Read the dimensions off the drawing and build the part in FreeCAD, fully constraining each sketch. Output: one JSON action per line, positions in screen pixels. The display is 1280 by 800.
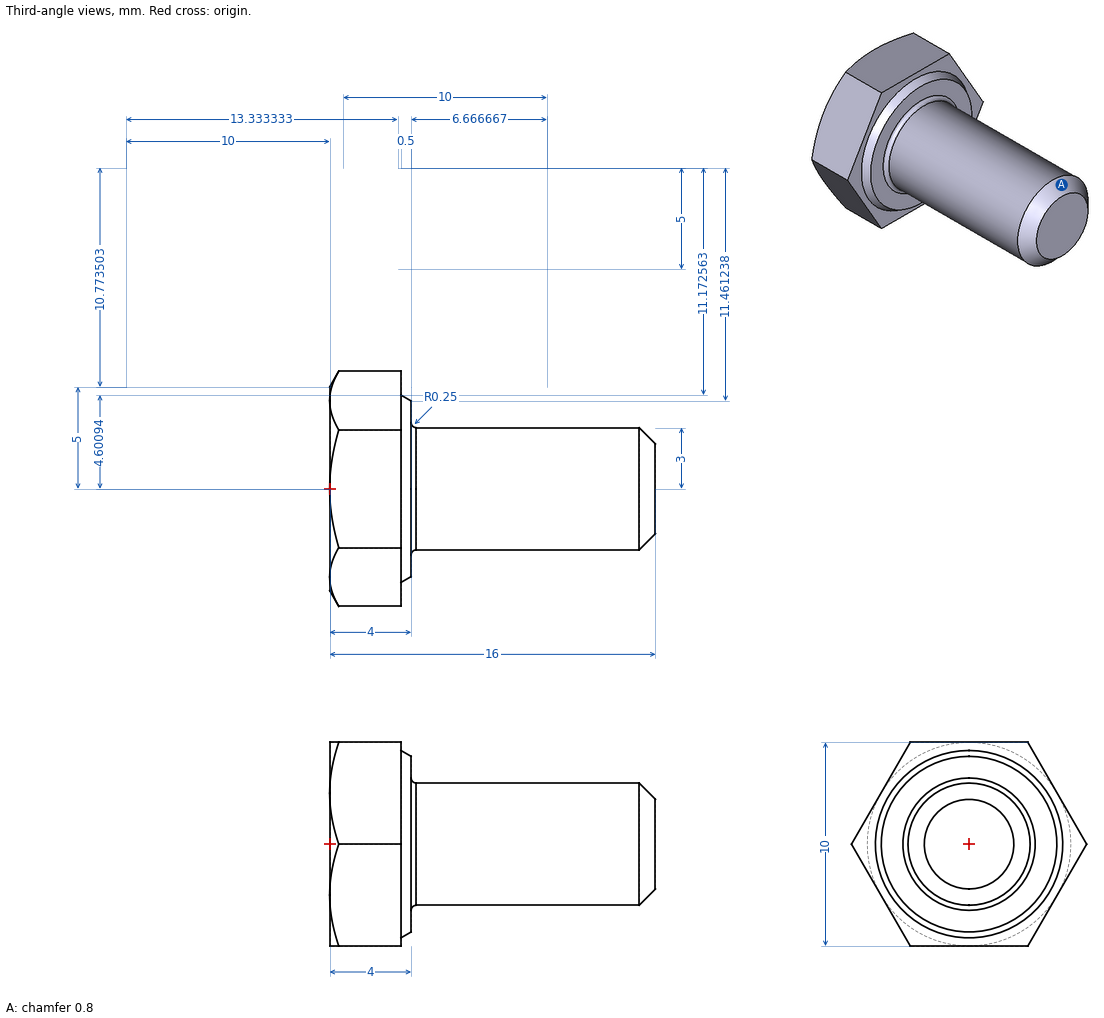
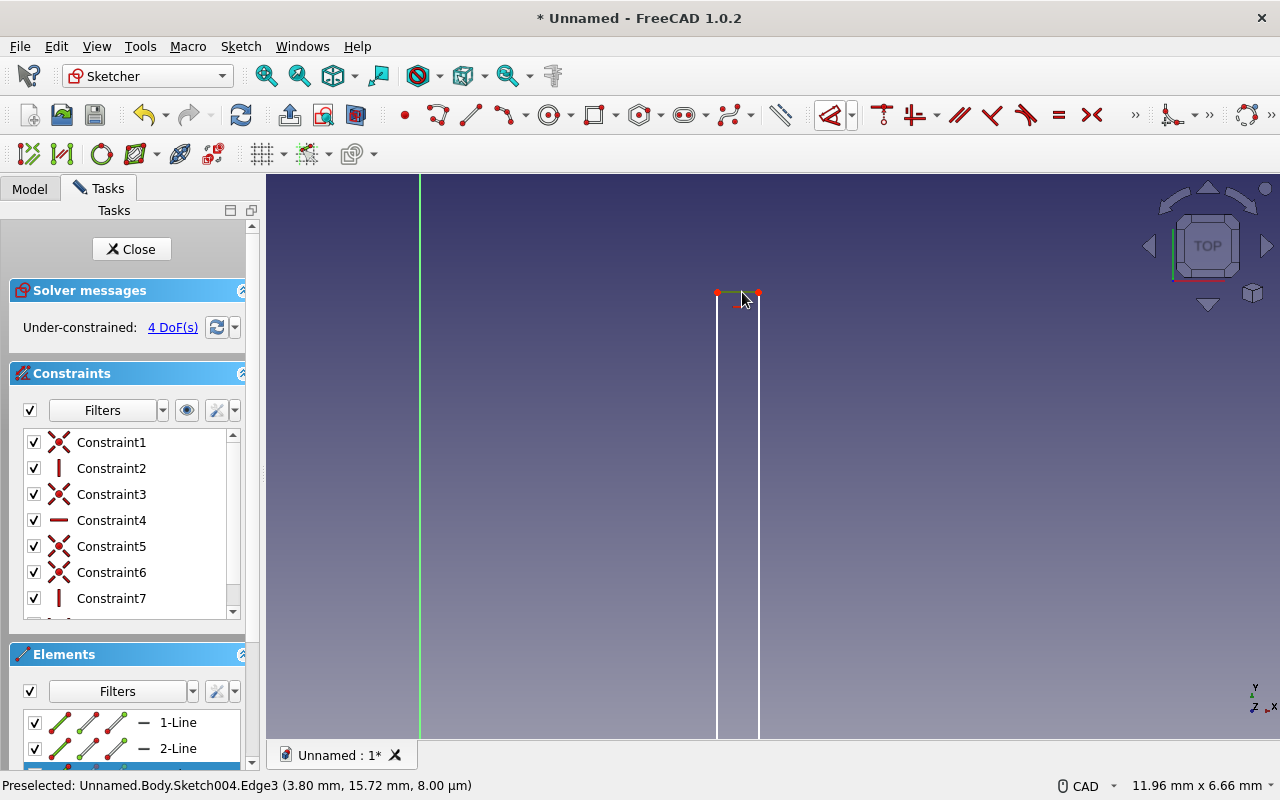
{"action": "left_click", "coordinate": [852, 116]}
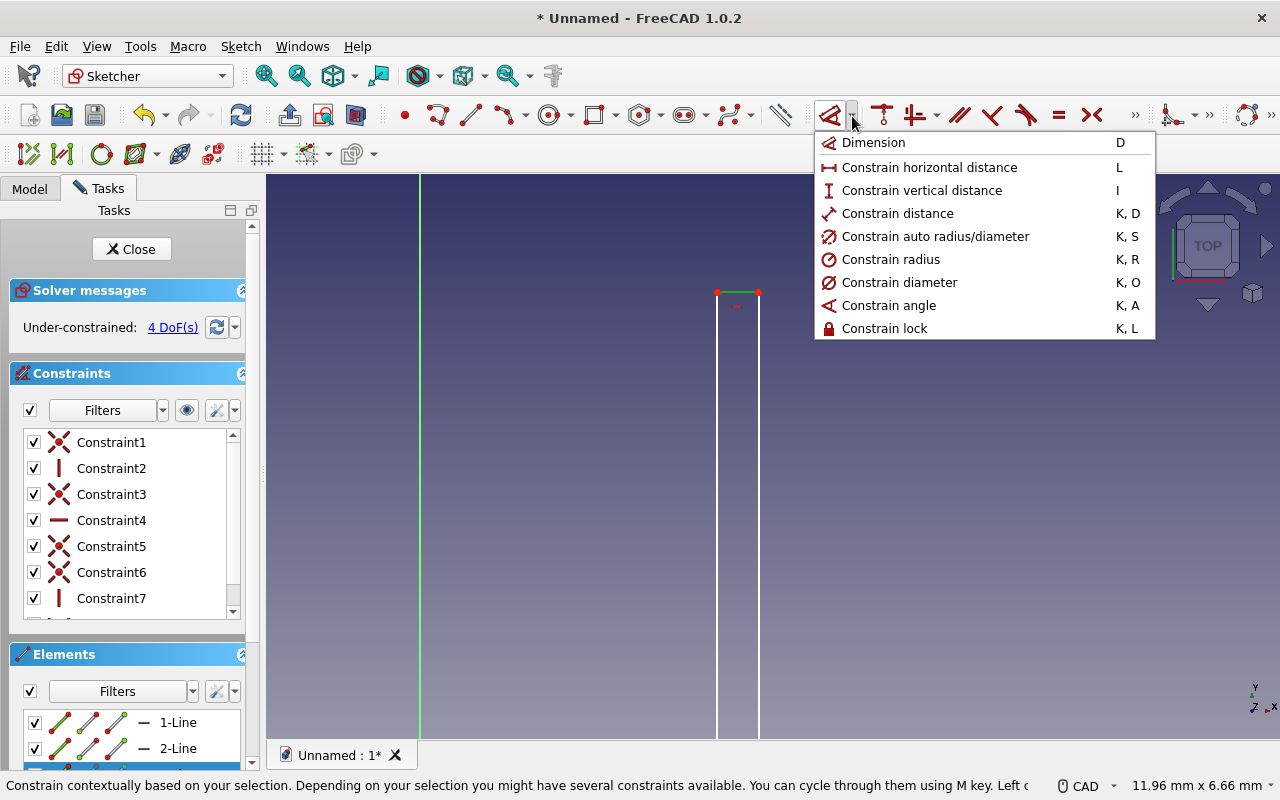
{"action": "left_click", "coordinate": [985, 168]}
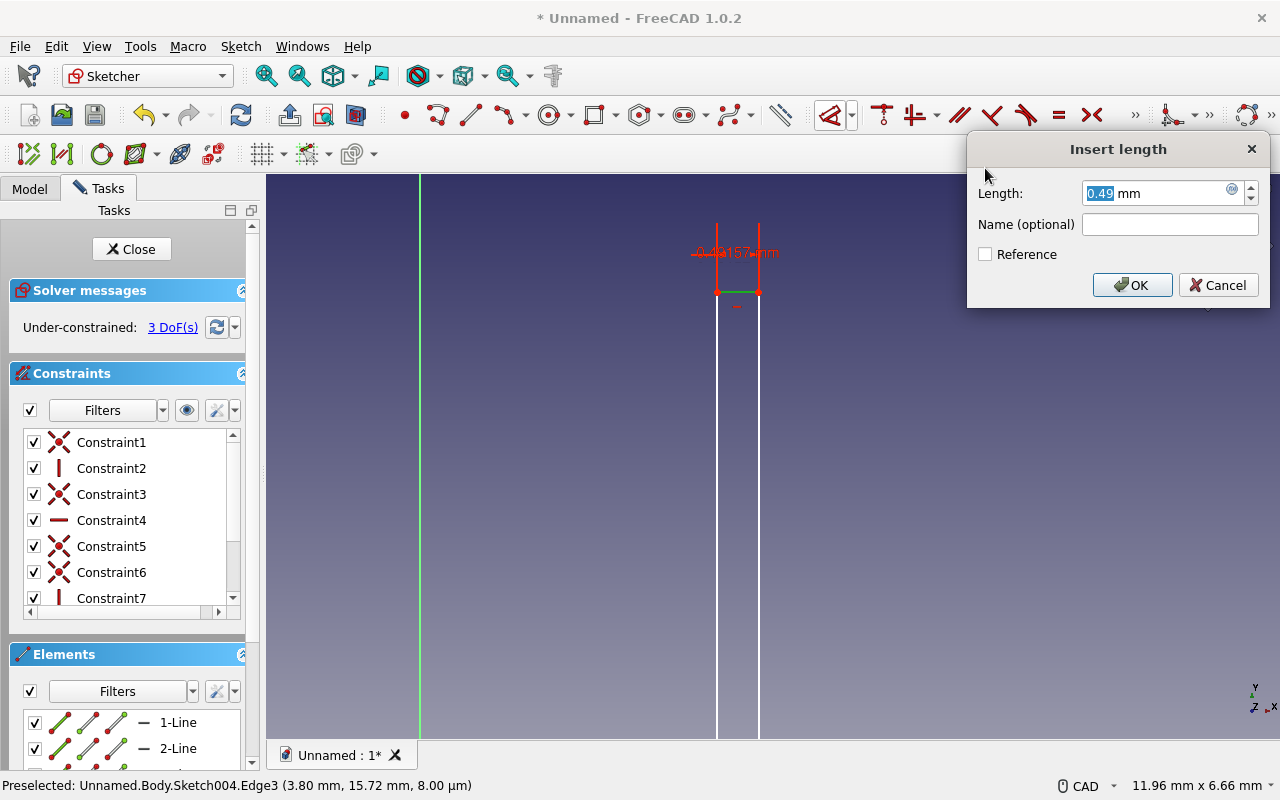
{"action": "type", "text": "0.5"}
{"action": "key", "text": "Return"}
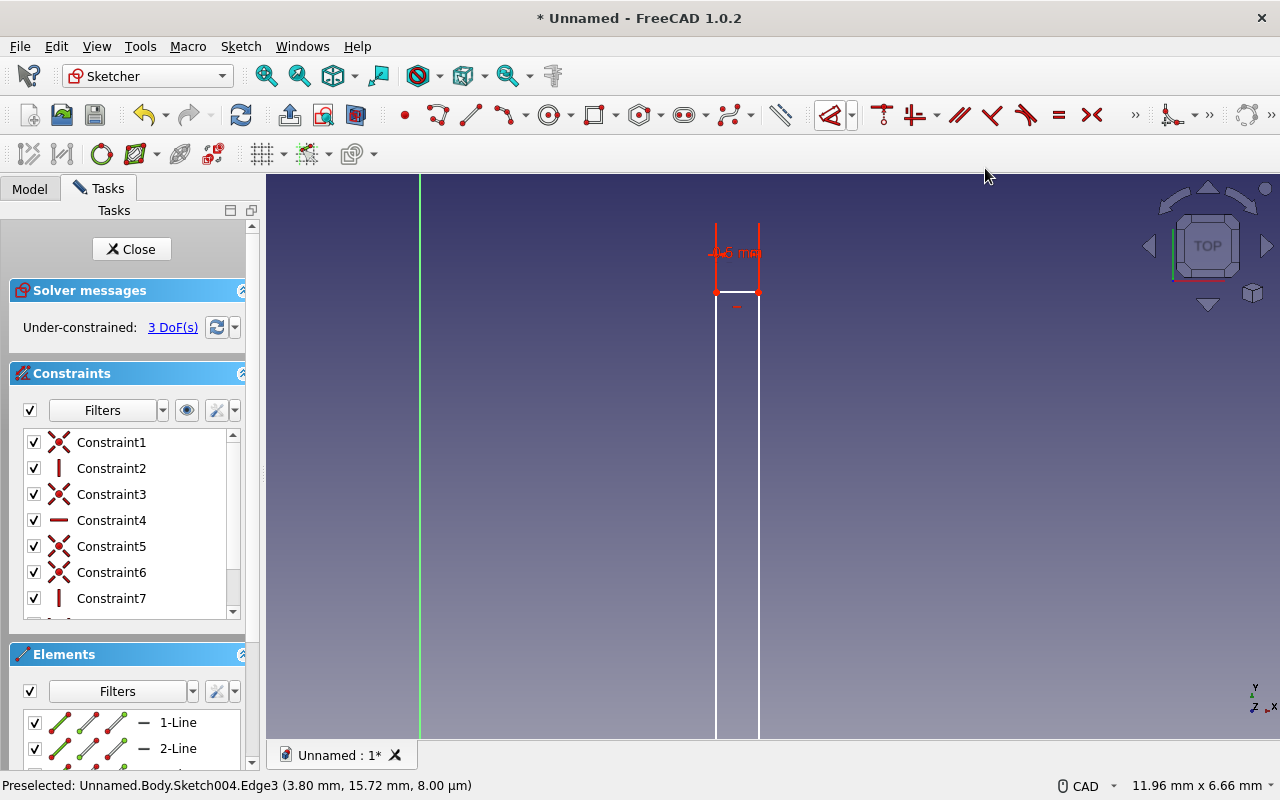
{"action": "scroll", "coordinate": [742, 293], "scroll_direction": "down", "scroll_amount": 7}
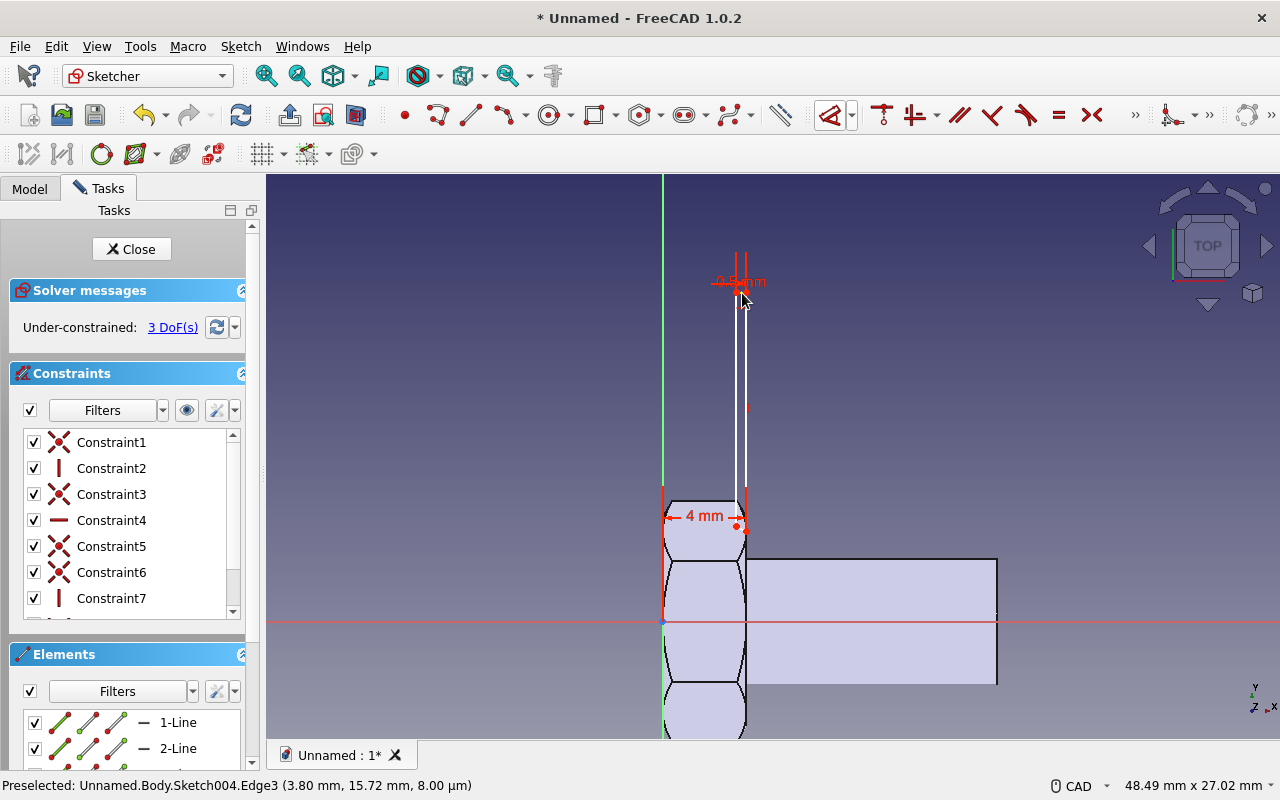
{"action": "left_click", "coordinate": [736, 527]}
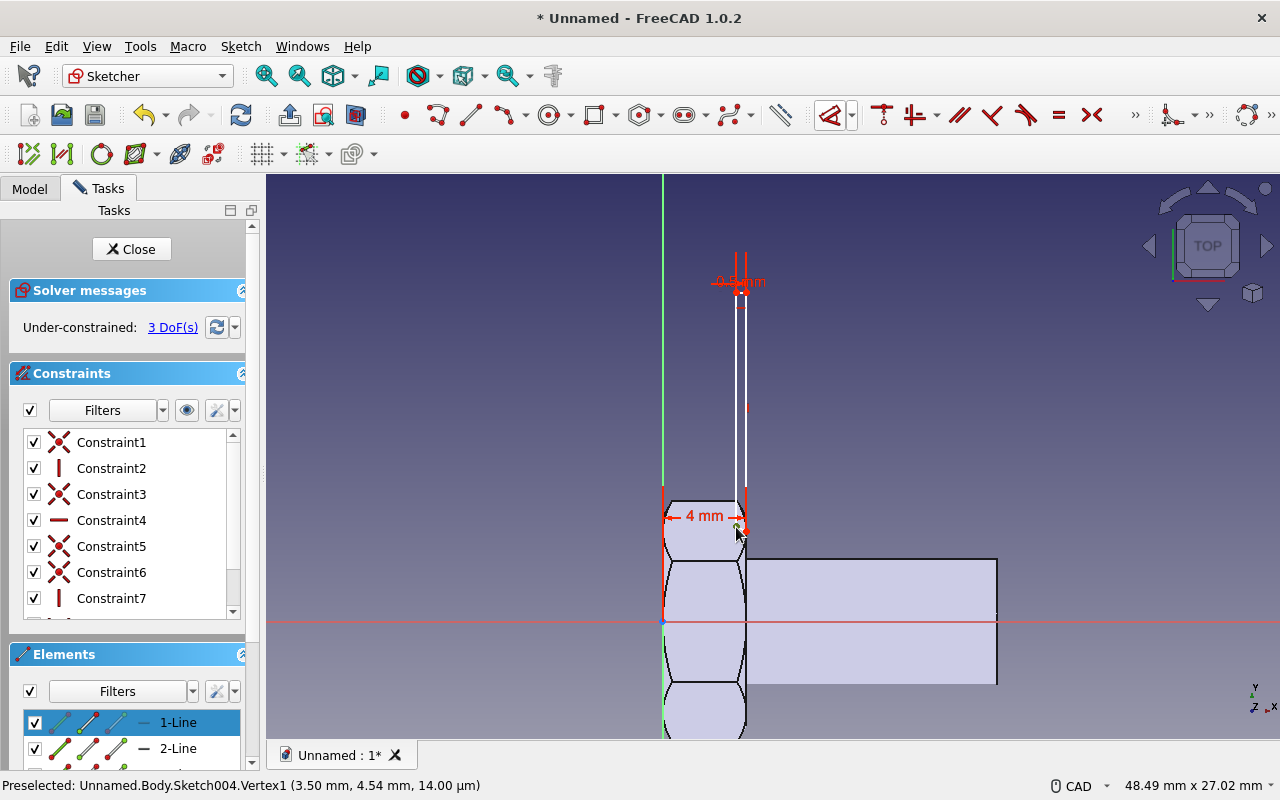
{"action": "left_click", "coordinate": [852, 116]}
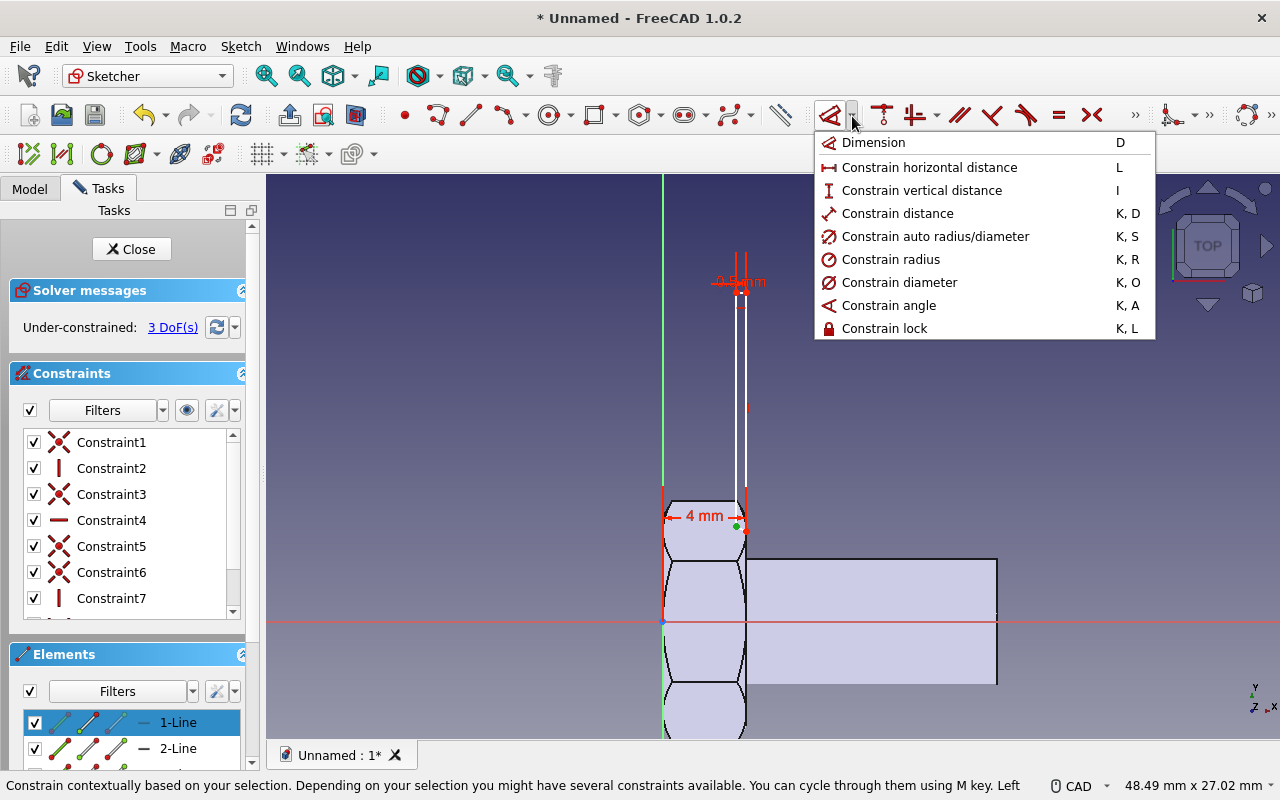
{"action": "left_click", "coordinate": [985, 190]}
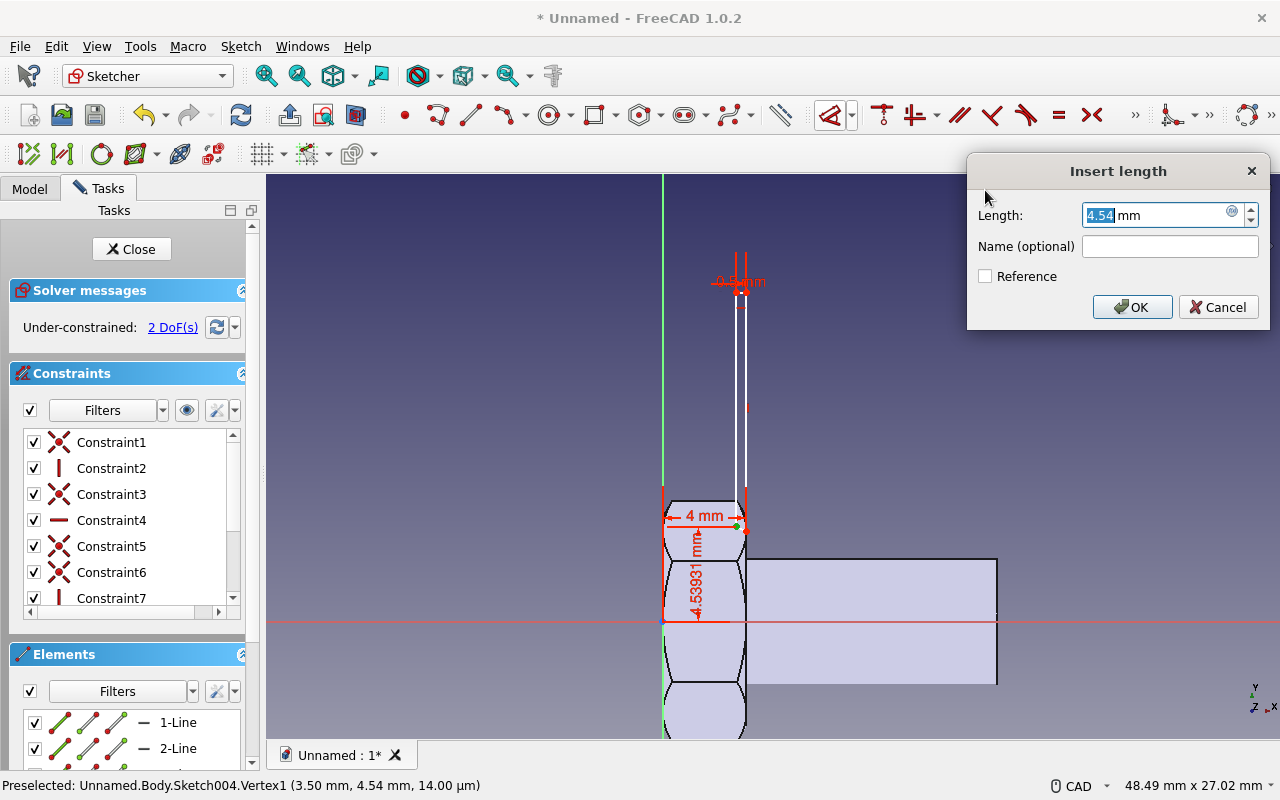
{"action": "type", "text": "4.60094"}
{"action": "key", "text": "Return"}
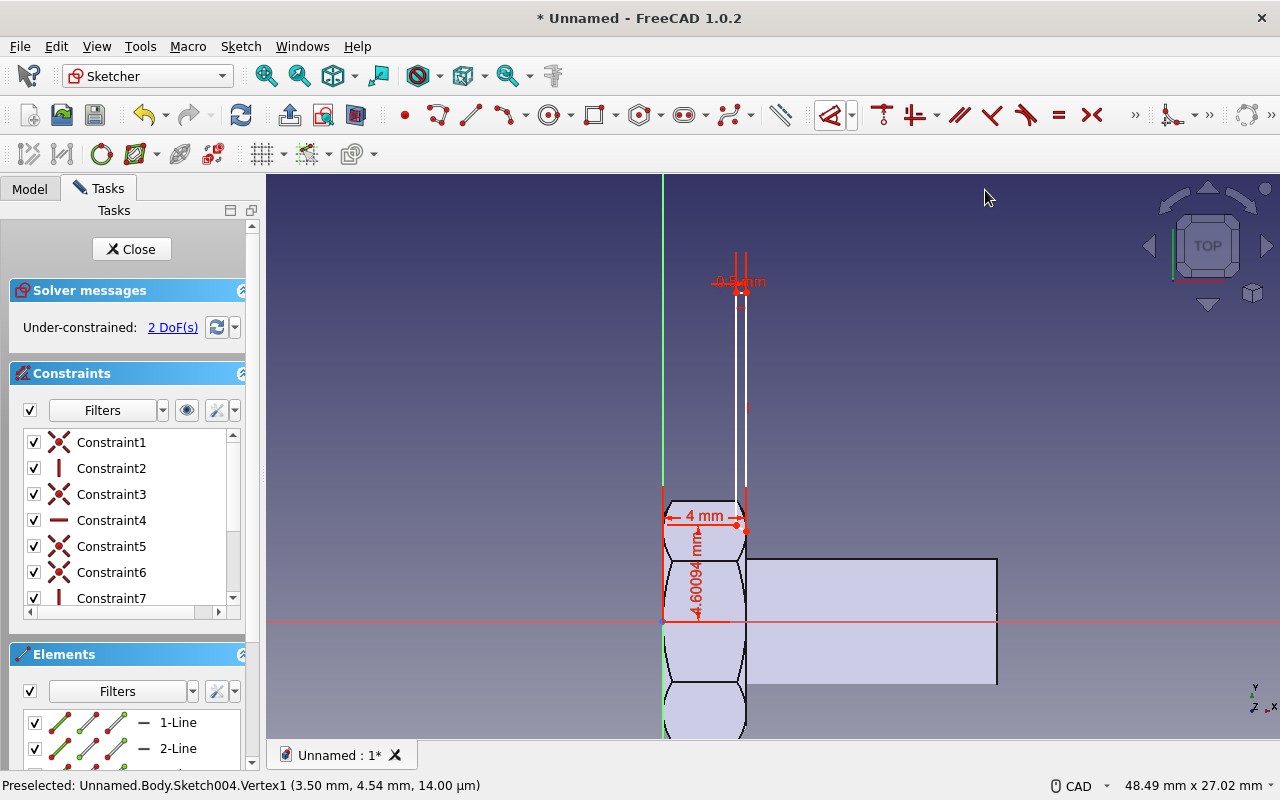
{"action": "scroll", "coordinate": [746, 460], "scroll_direction": "up", "scroll_amount": 2}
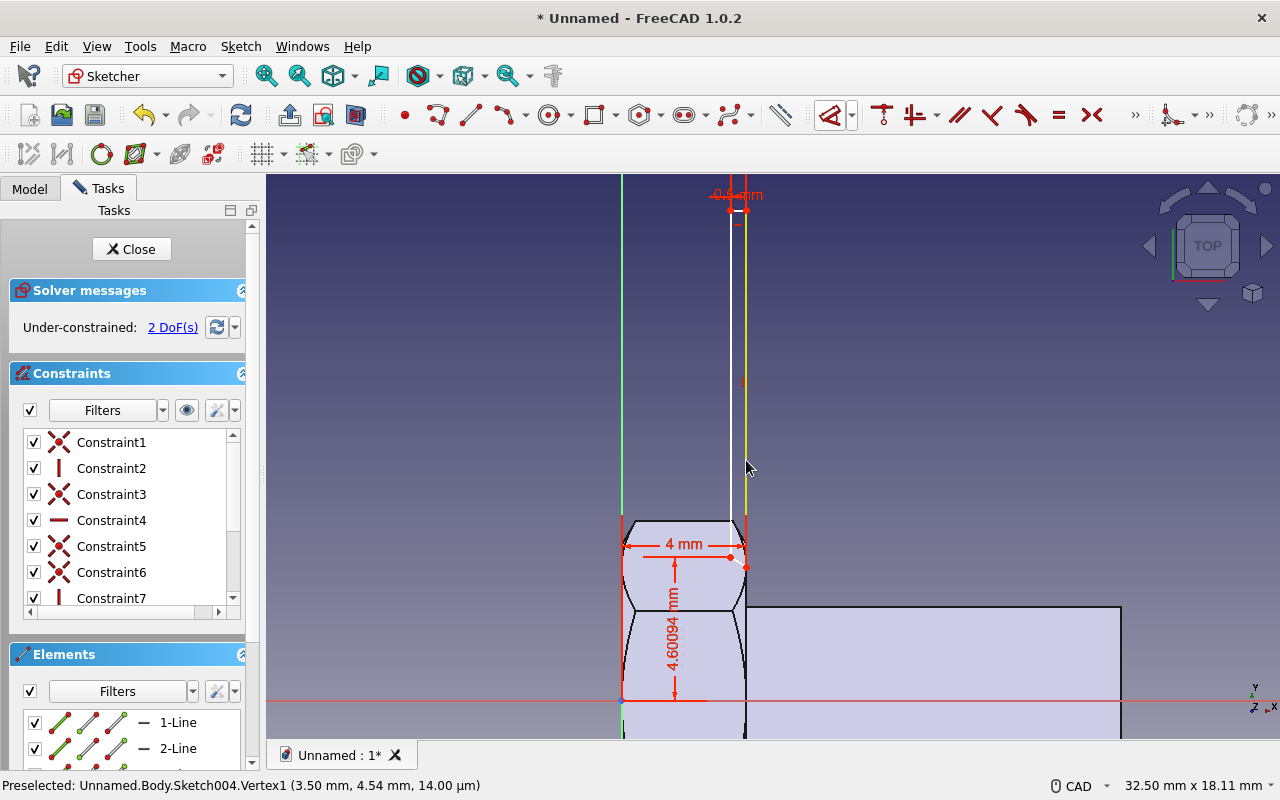
{"action": "left_click", "coordinate": [746, 460]}